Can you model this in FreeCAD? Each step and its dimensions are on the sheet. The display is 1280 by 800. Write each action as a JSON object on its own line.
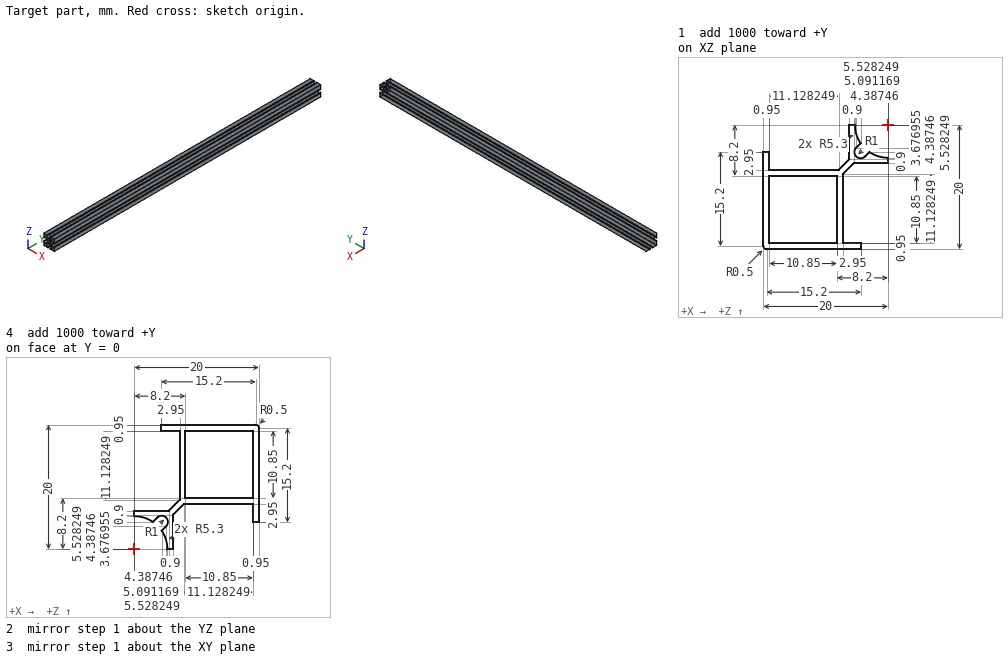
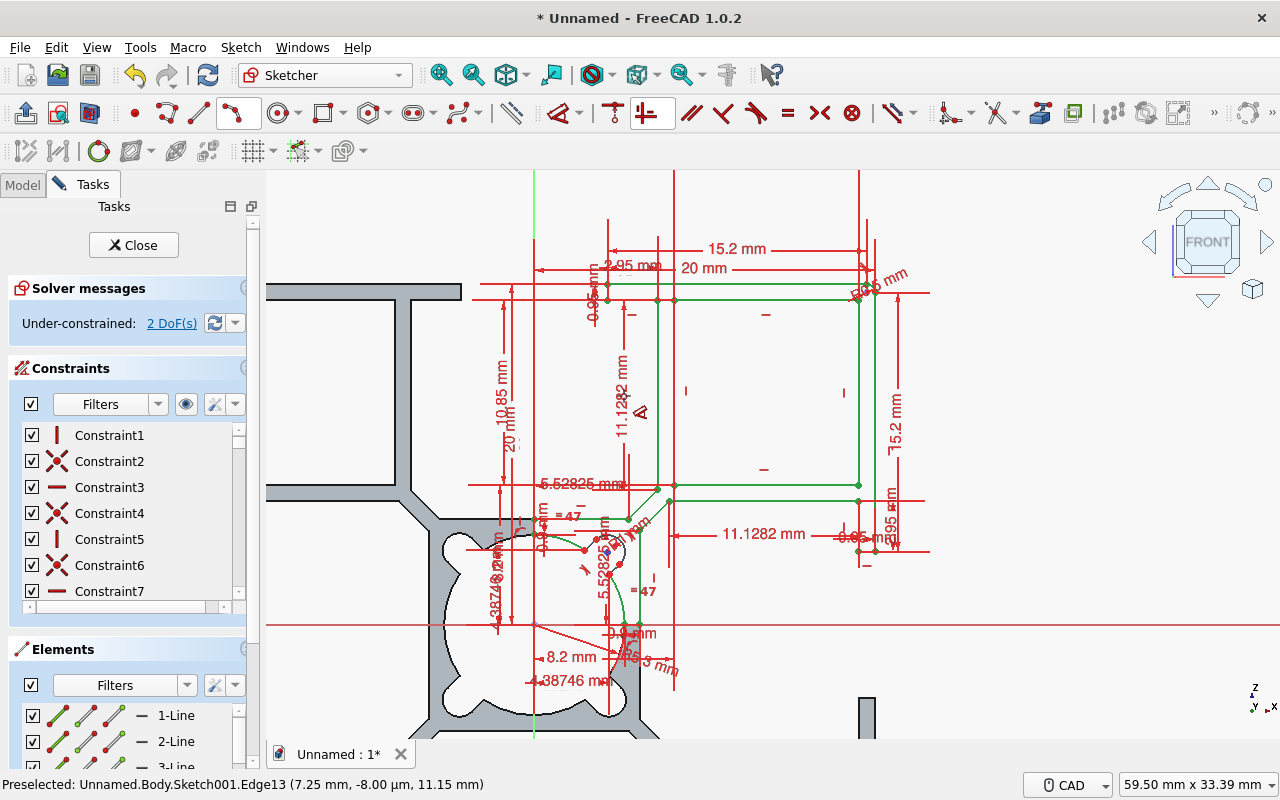
{"action": "left_click", "coordinate": [619, 565]}
{"action": "left_click", "coordinate": [577, 707]}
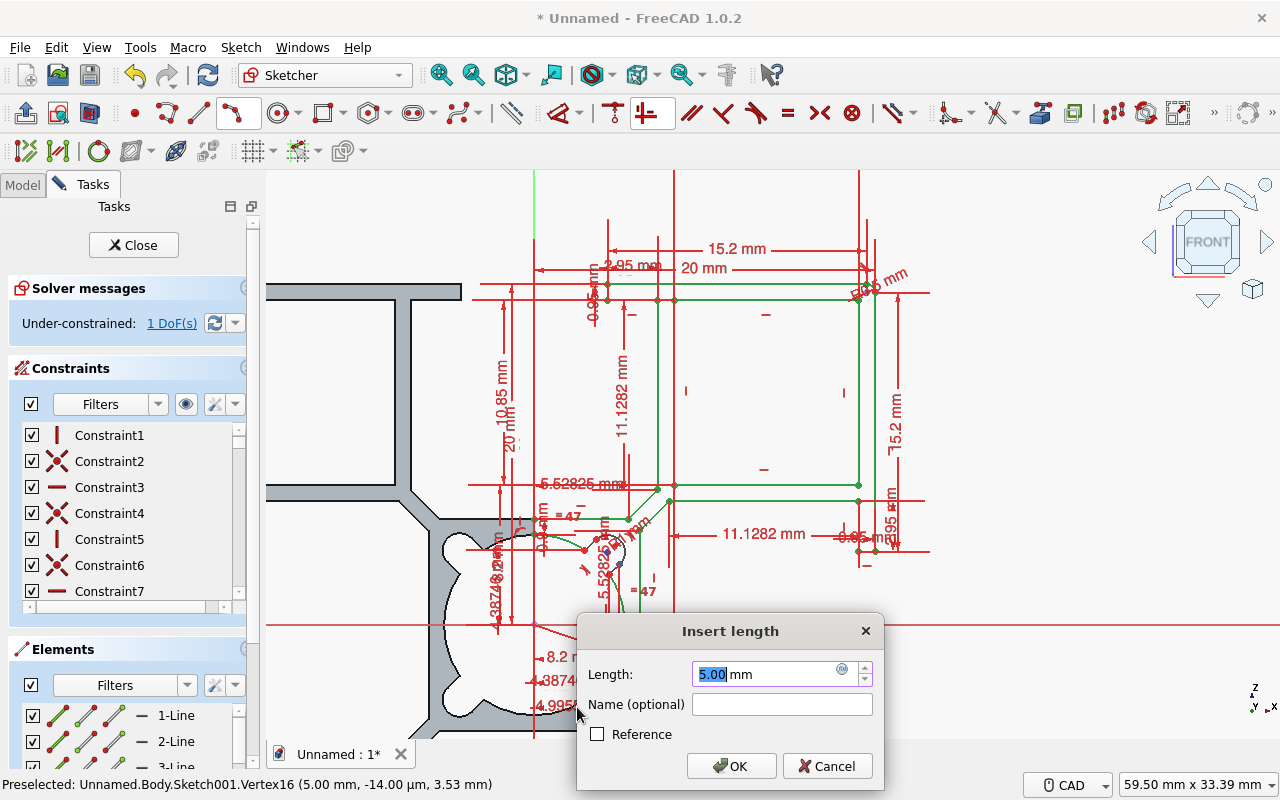
{"action": "type", "text": "5.091169"}
{"action": "key", "text": "Return"}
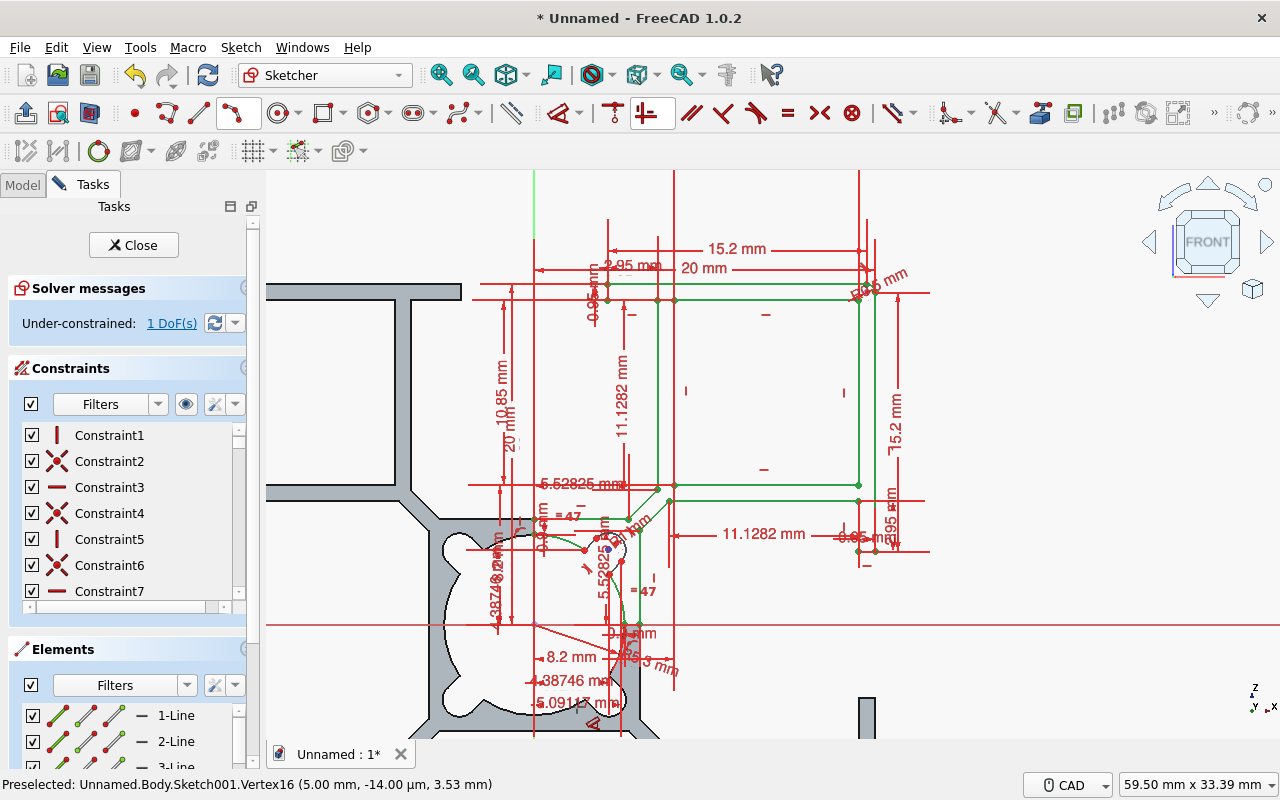
{"action": "left_click", "coordinate": [621, 562]}
{"action": "left_click", "coordinate": [655, 593]}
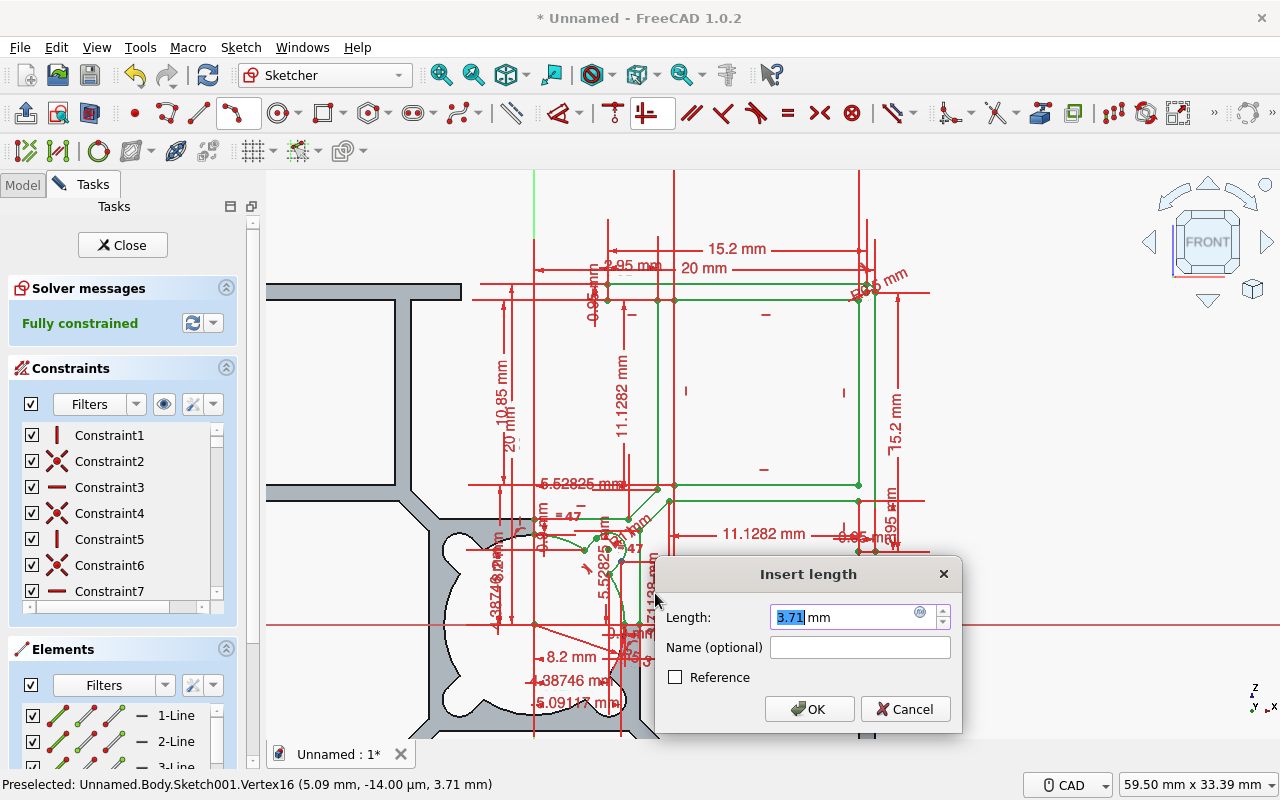
{"action": "type", "text": "3.676955"}
{"action": "key", "text": "Return"}
{"action": "key", "text": "Escape"}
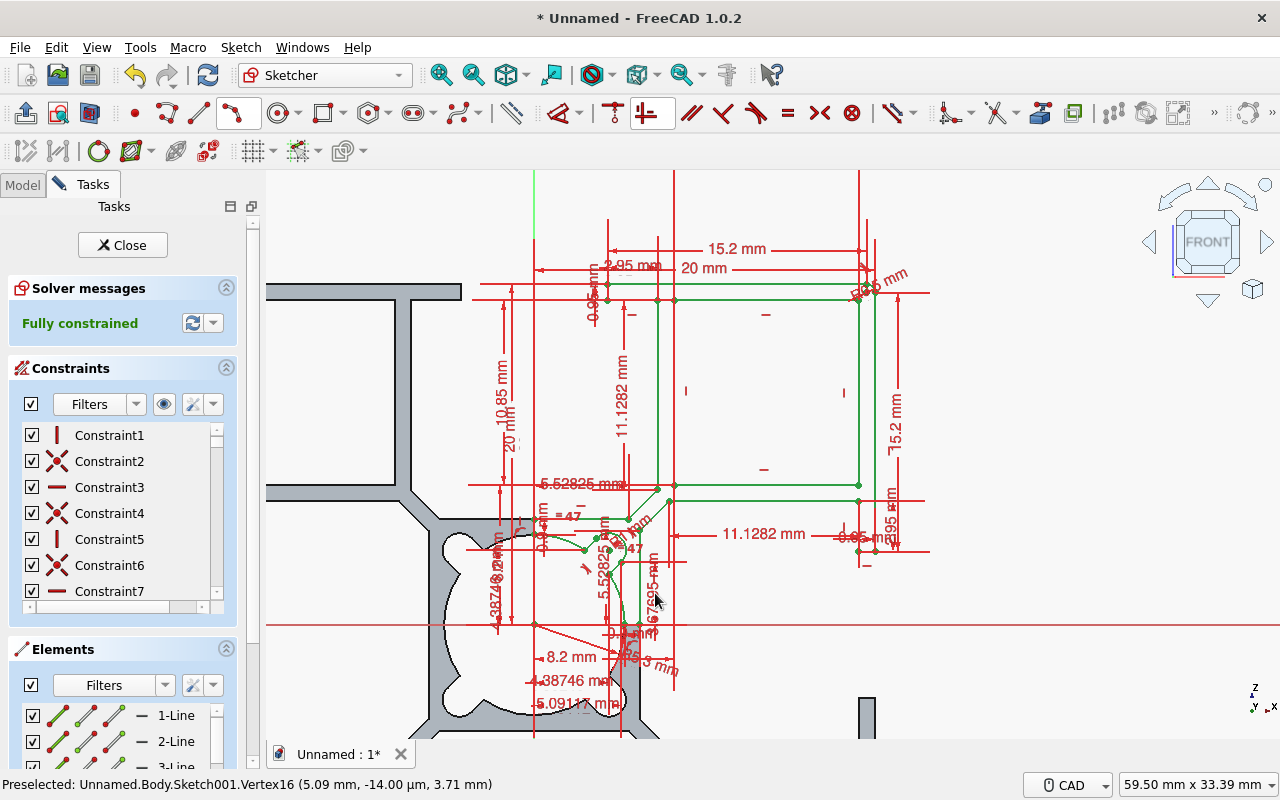
{"action": "left_click", "coordinate": [123, 245]}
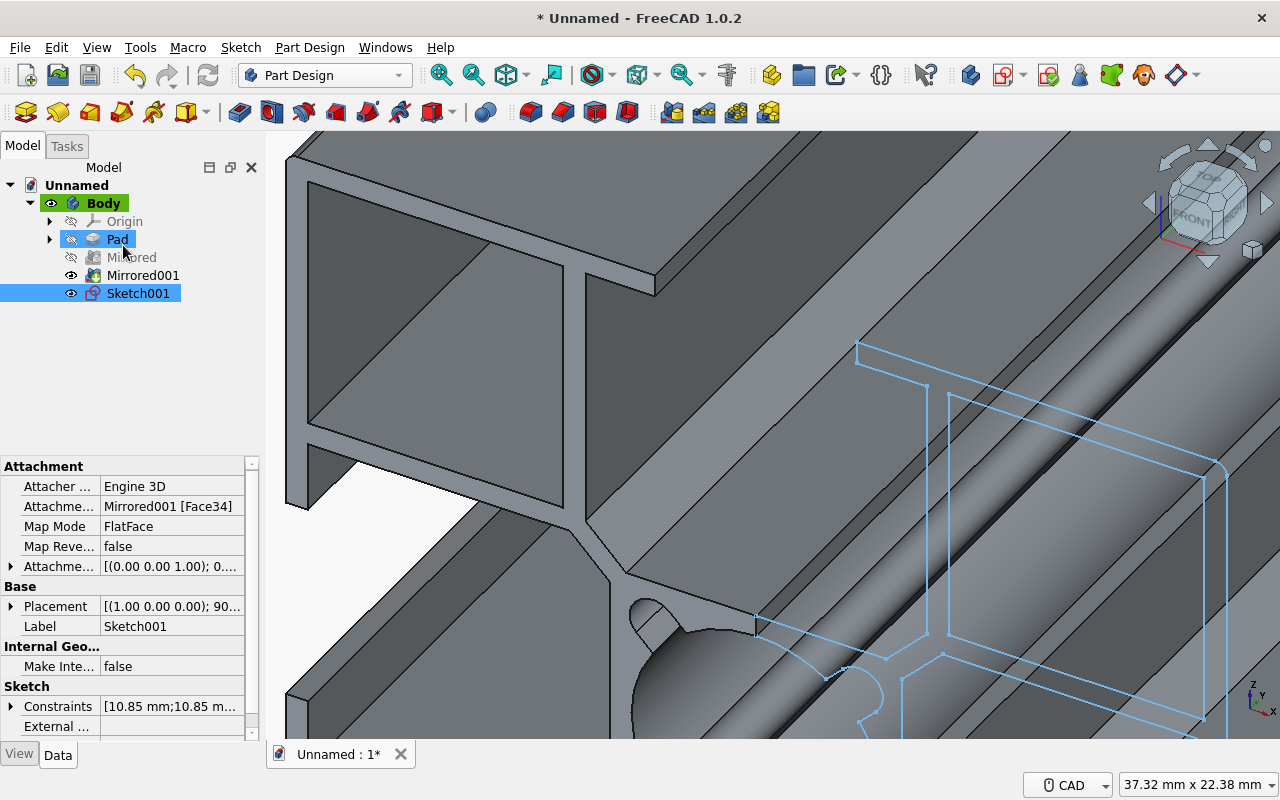
{"action": "left_click", "coordinate": [26, 112]}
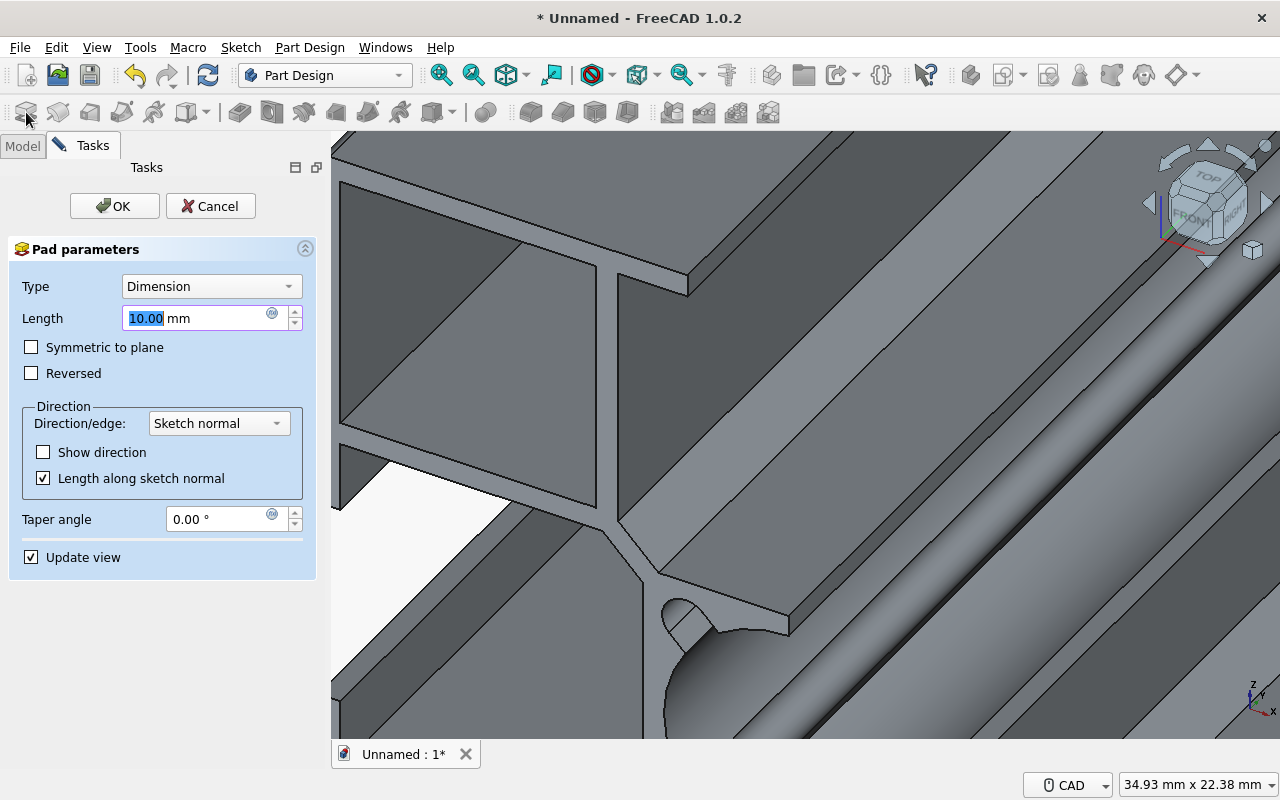
{"action": "type", "text": "1000"}
{"action": "key", "text": "Tab"}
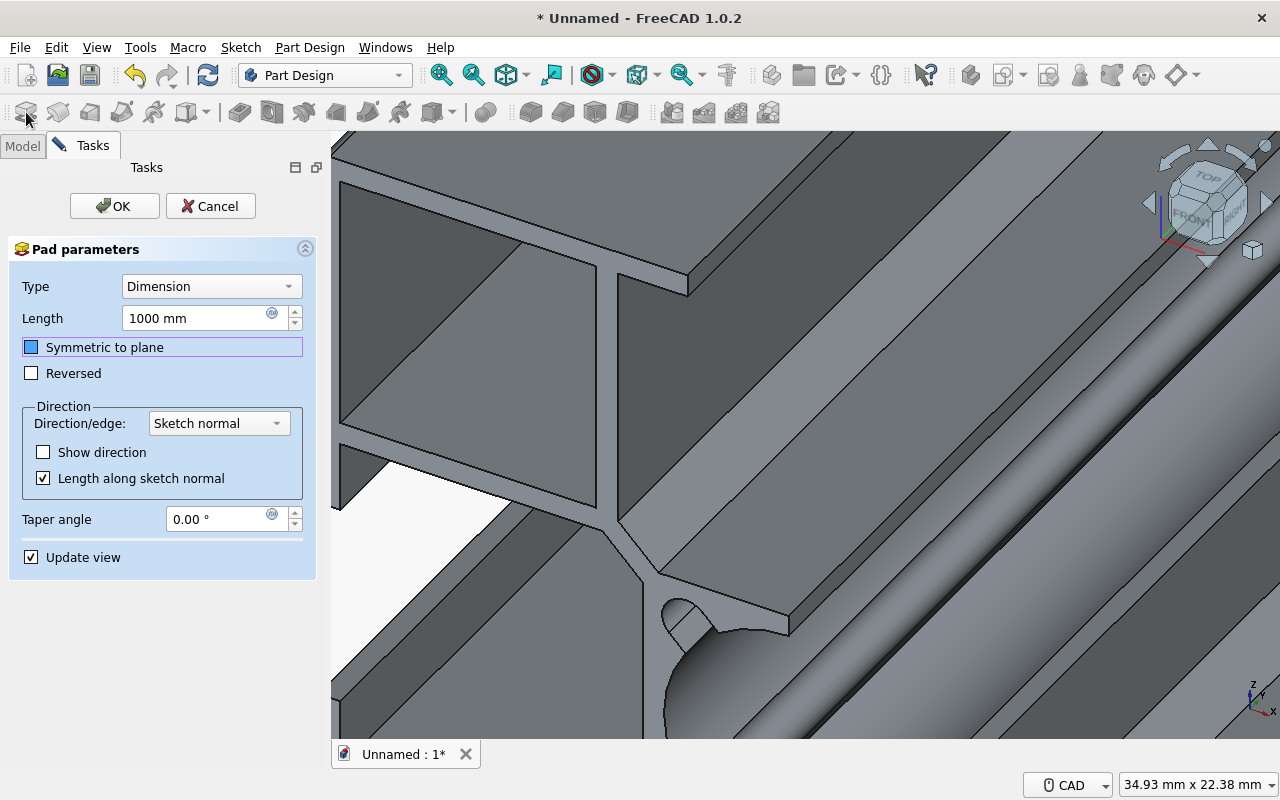
{"action": "left_click", "coordinate": [30, 373]}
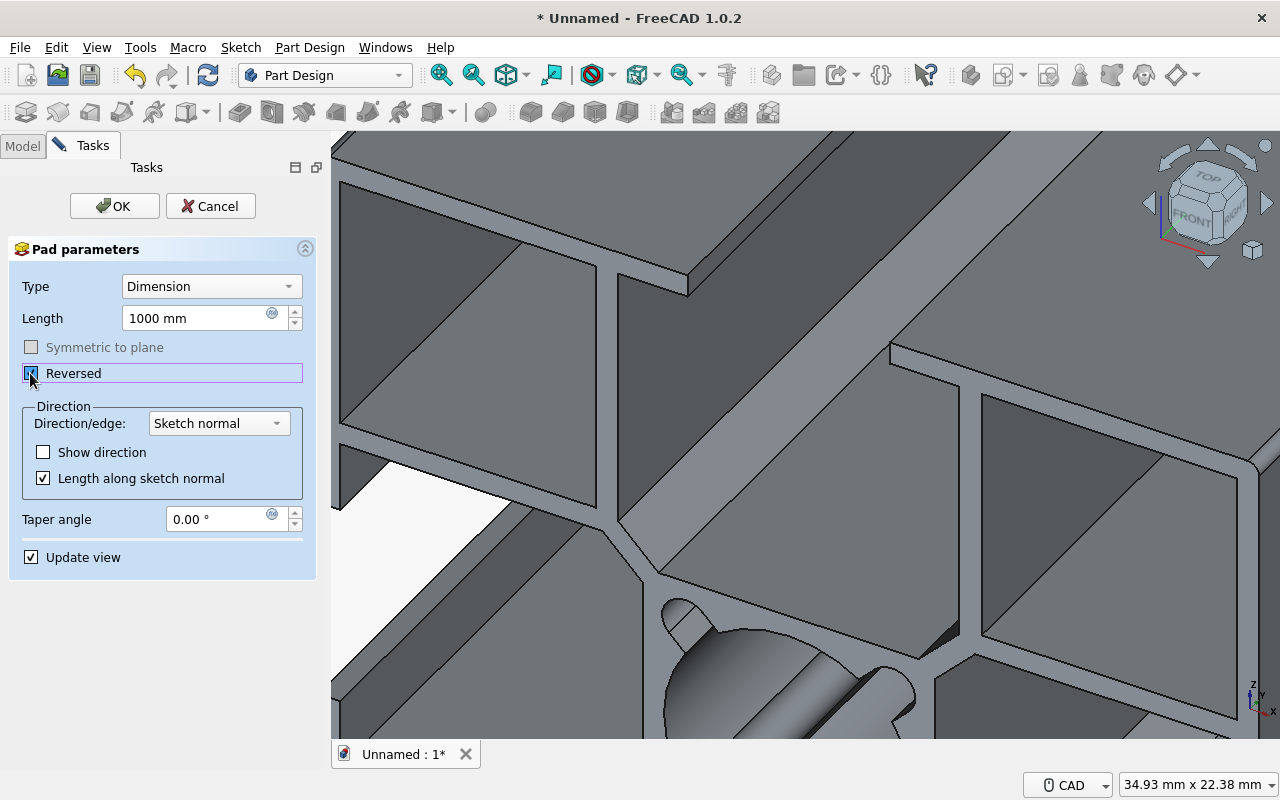
{"action": "left_click", "coordinate": [115, 206]}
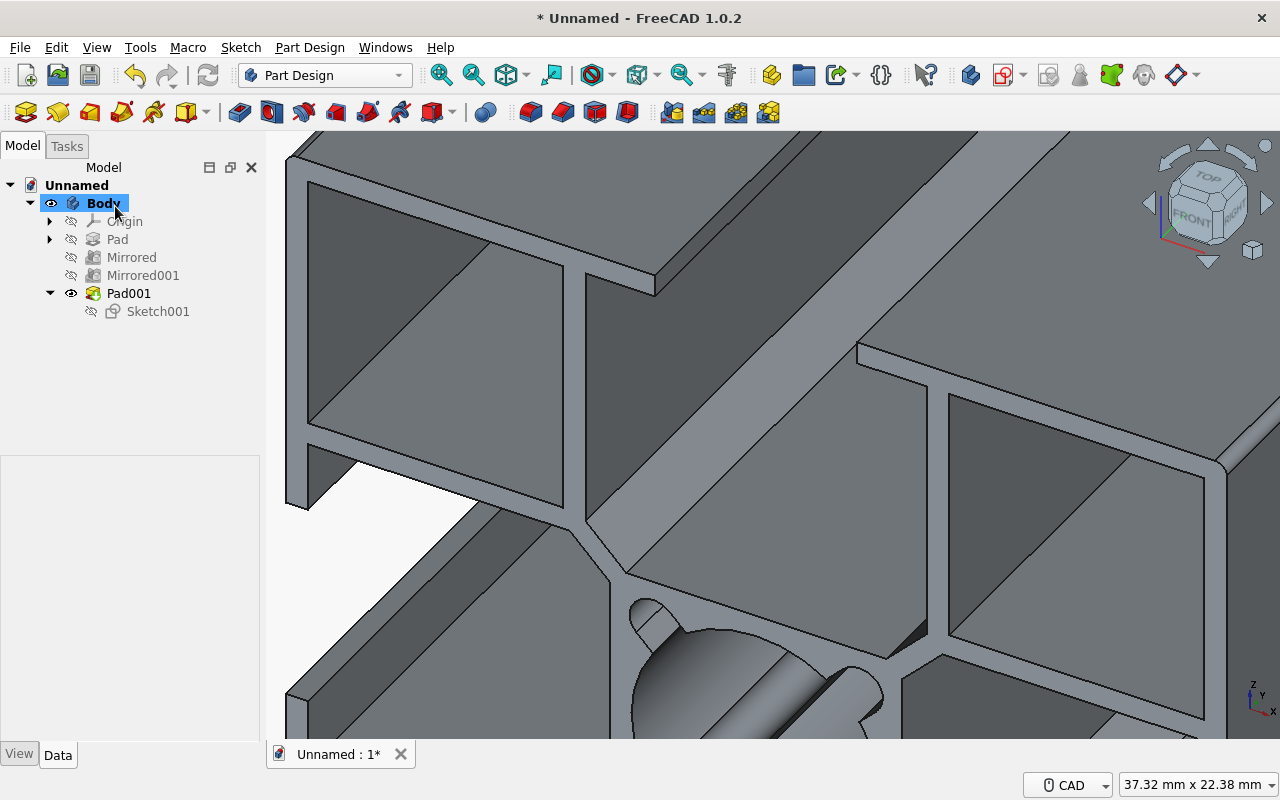
{"action": "key", "text": "0"}